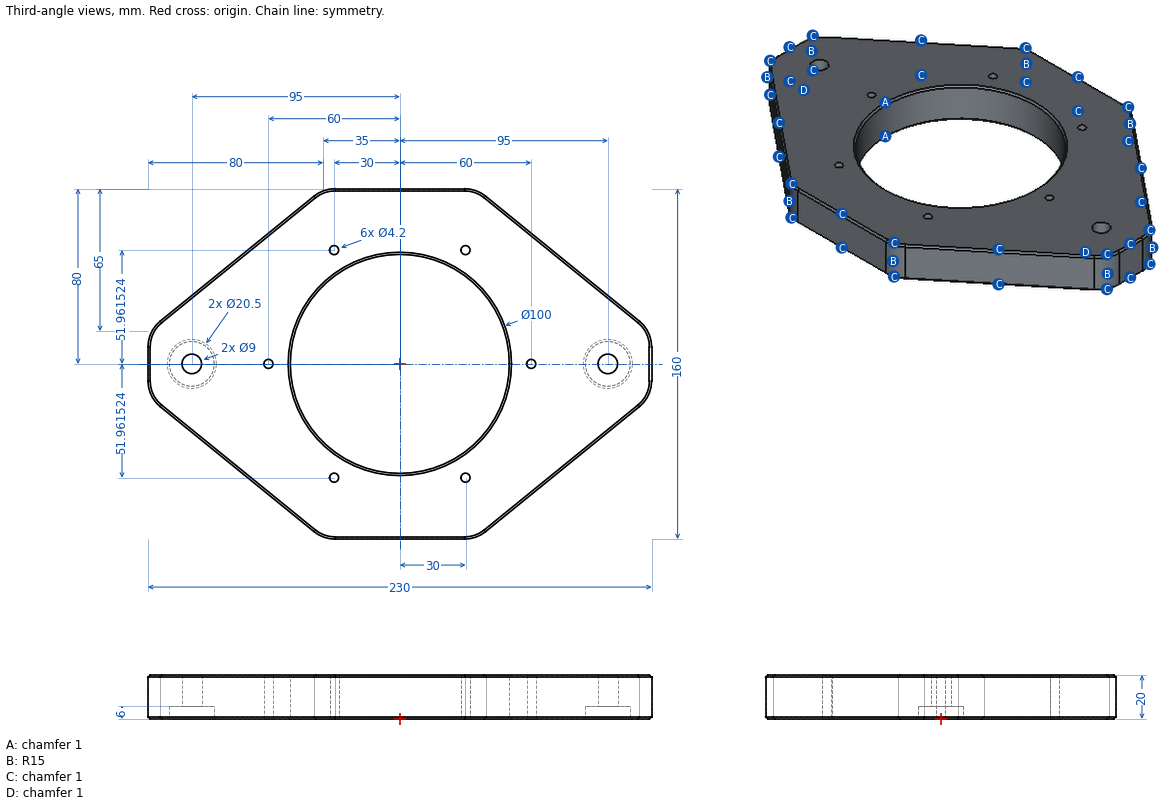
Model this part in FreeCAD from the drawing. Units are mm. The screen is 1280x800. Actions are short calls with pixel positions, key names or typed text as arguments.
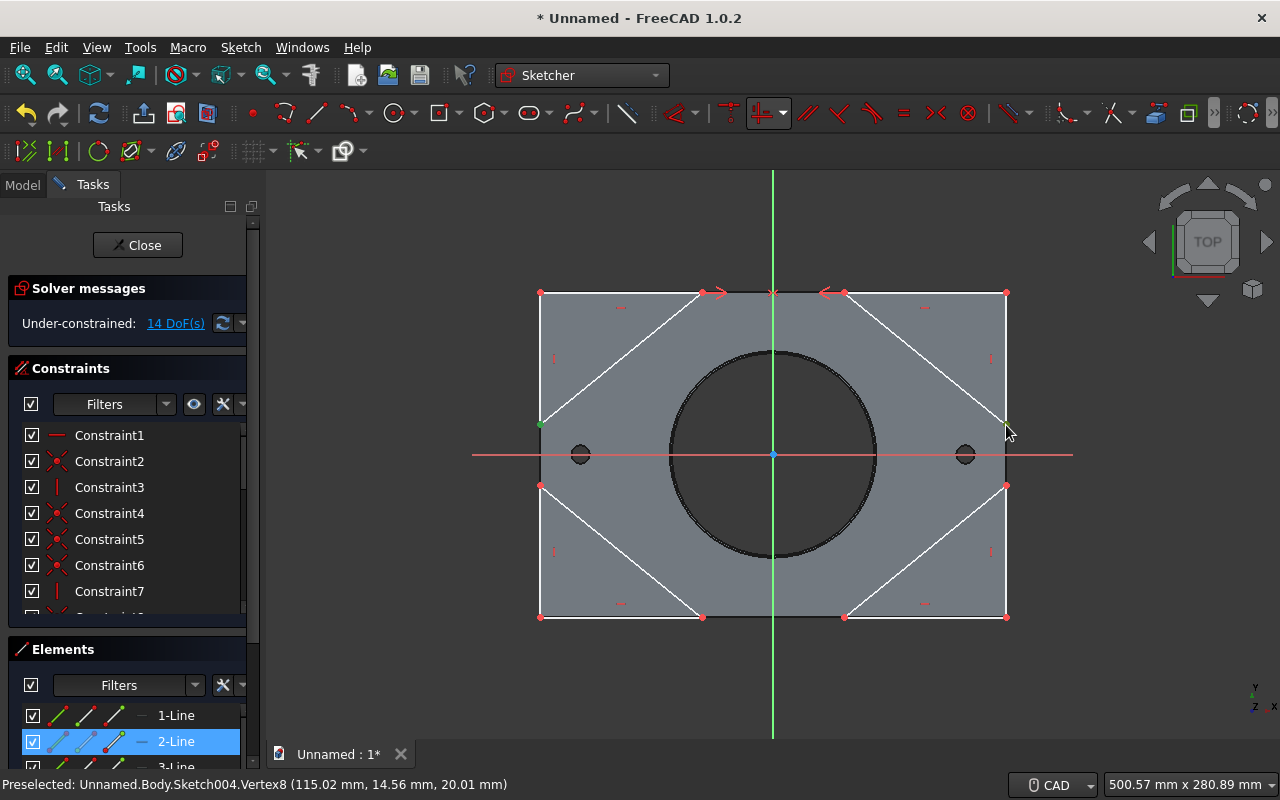
click(773, 674)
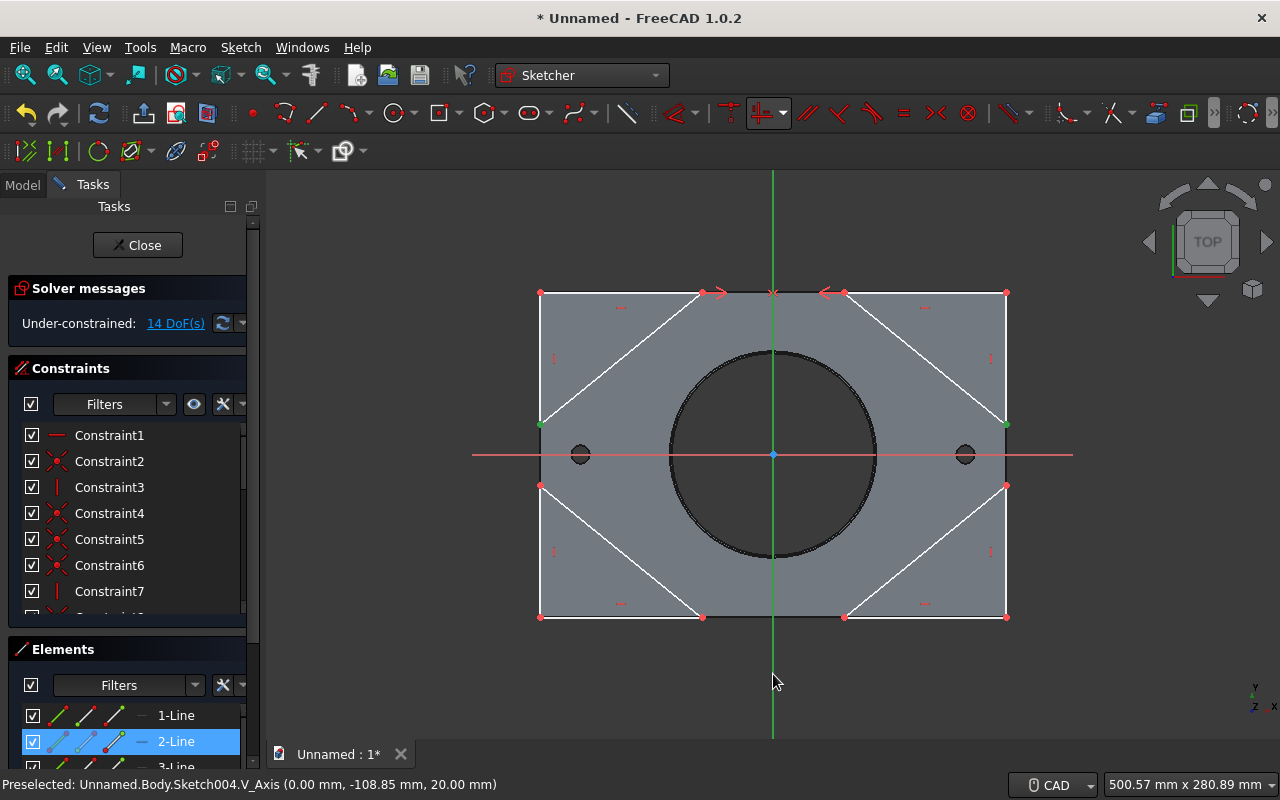
click(936, 114)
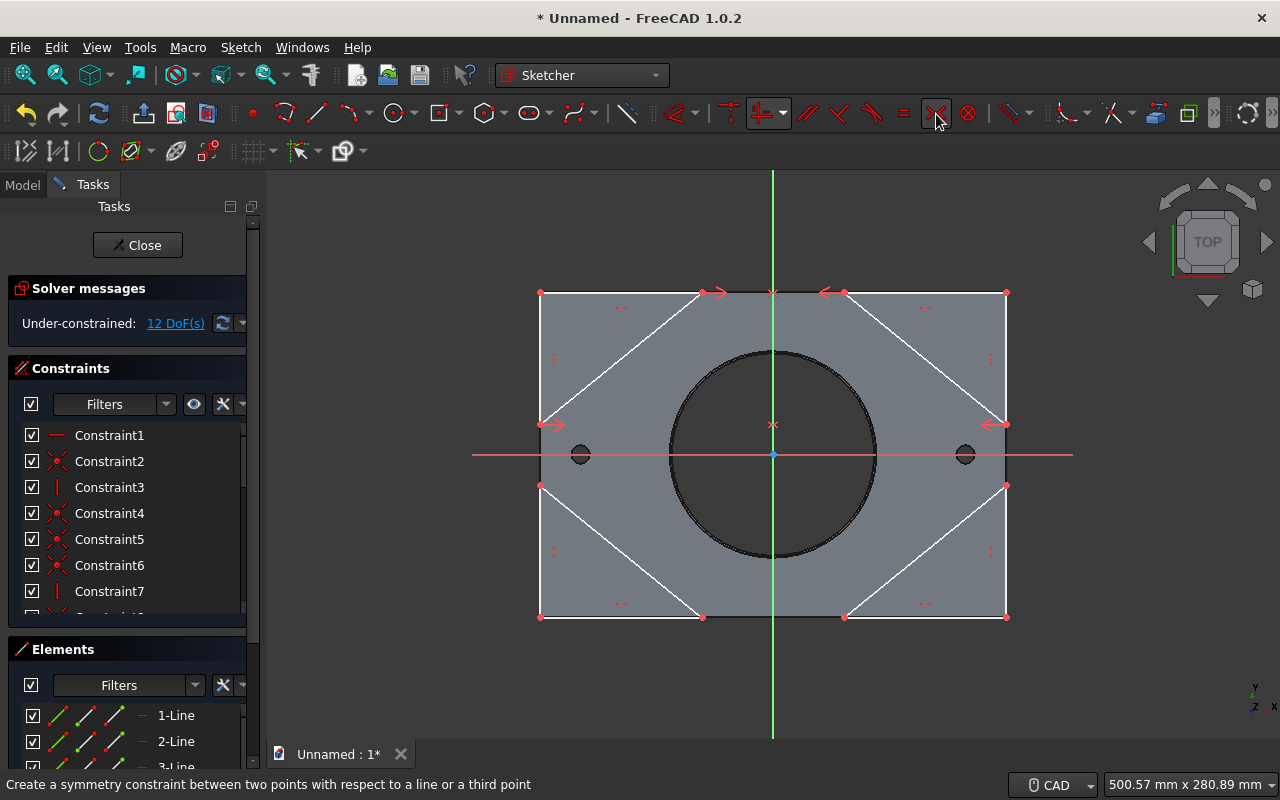
click(702, 293)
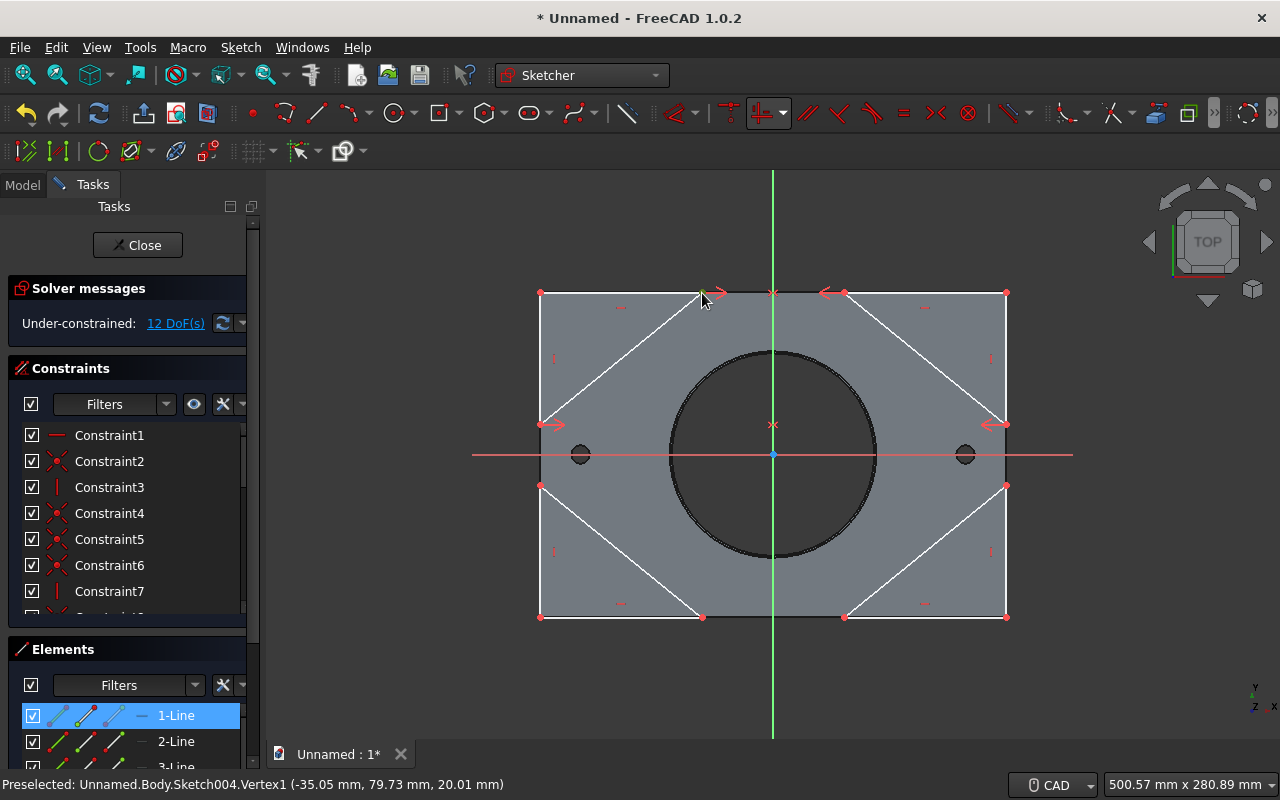
click(702, 618)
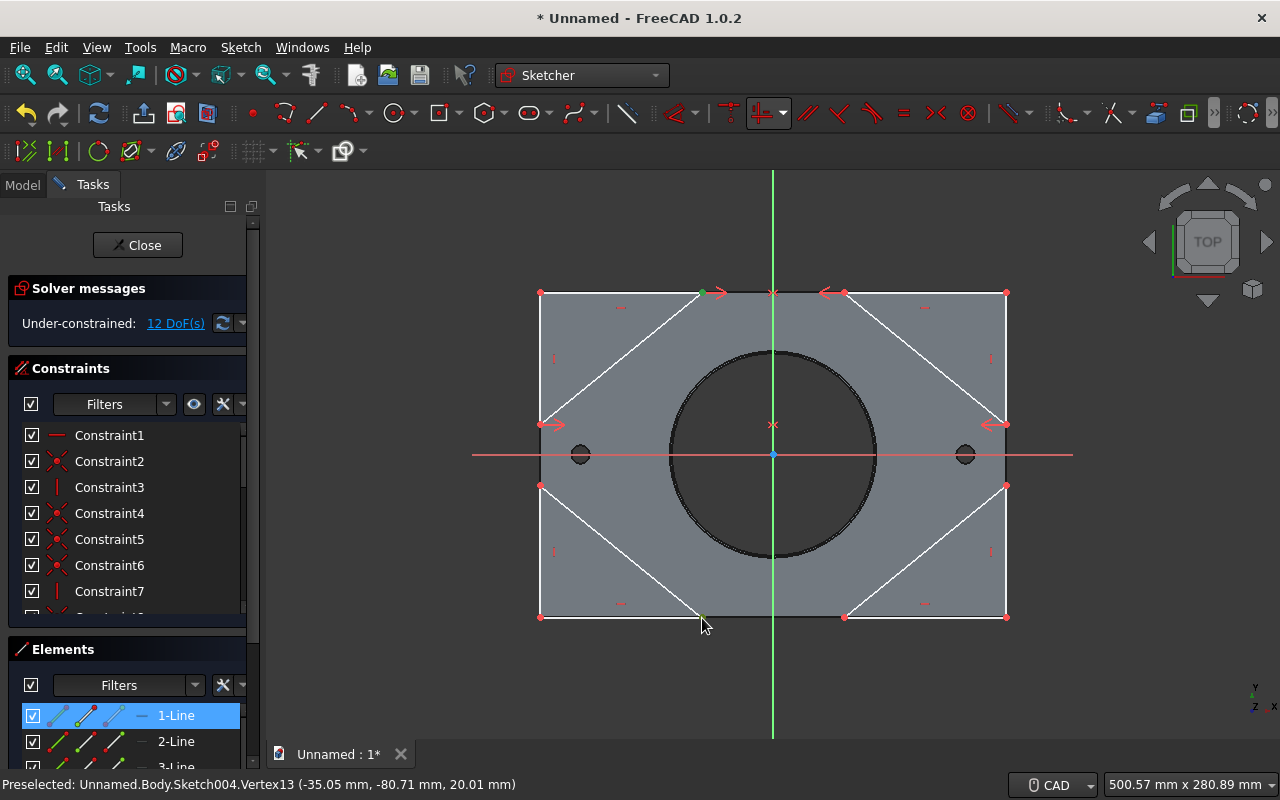
click(470, 454)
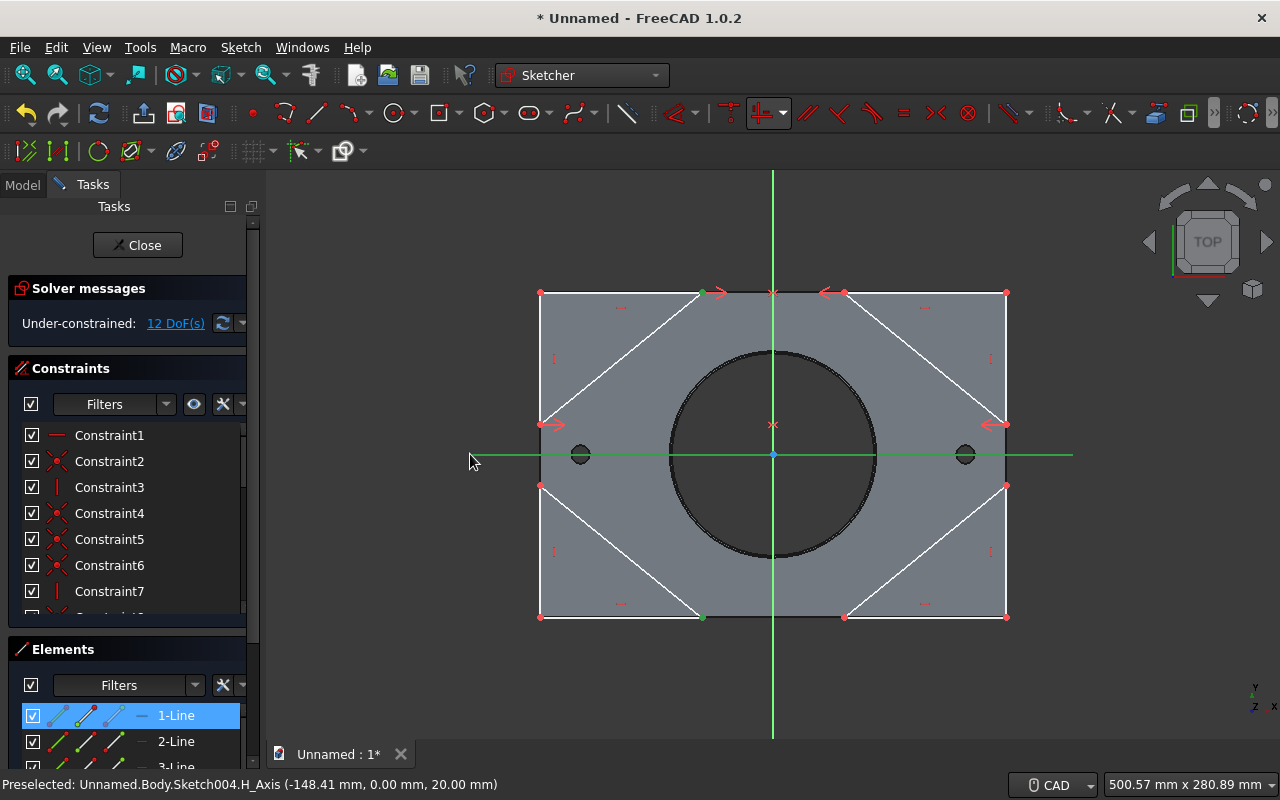
click(936, 114)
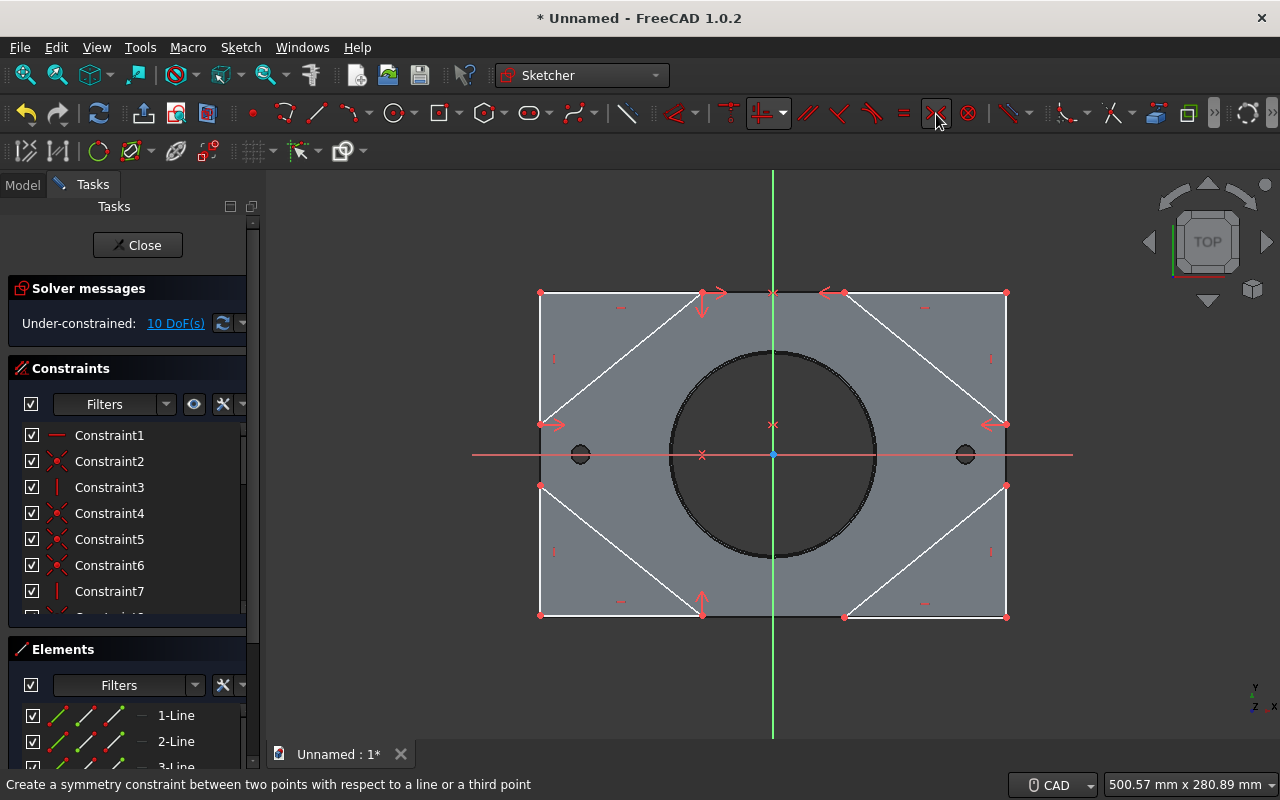
click(540, 425)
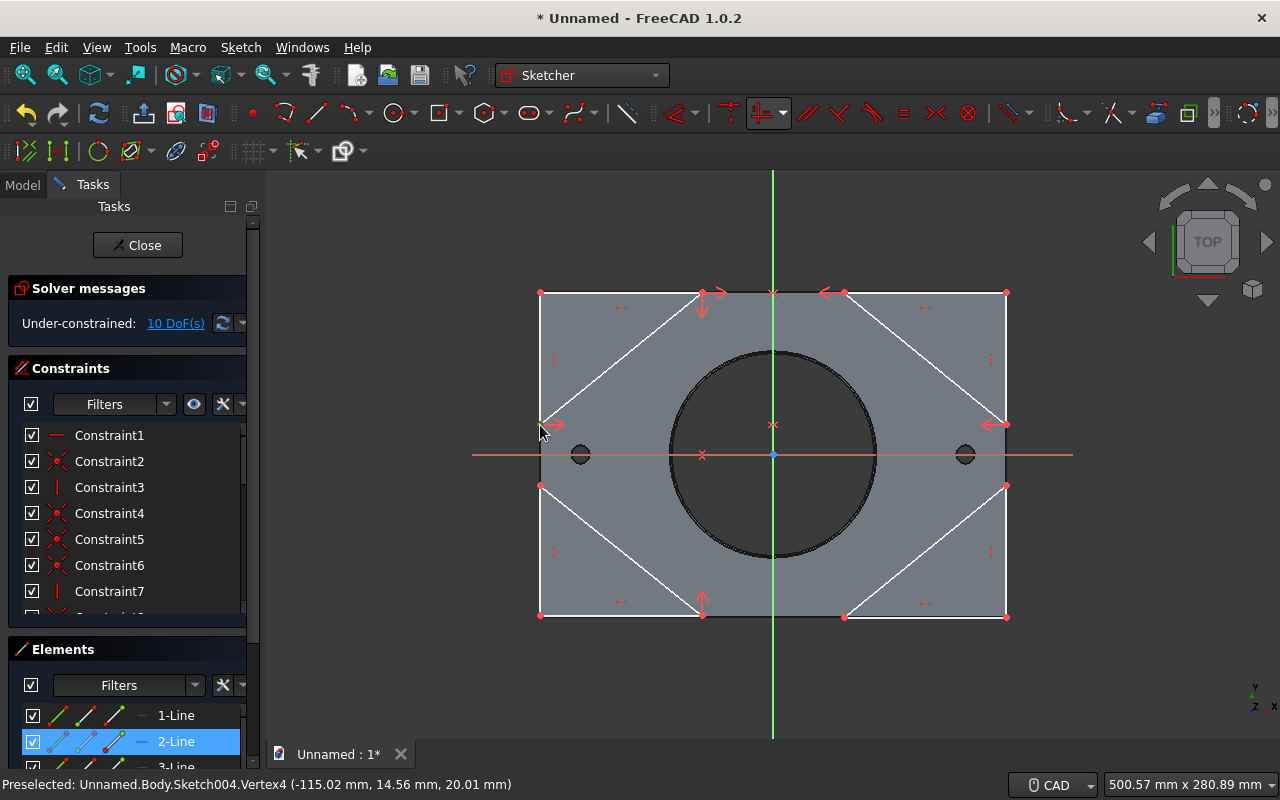
click(540, 486)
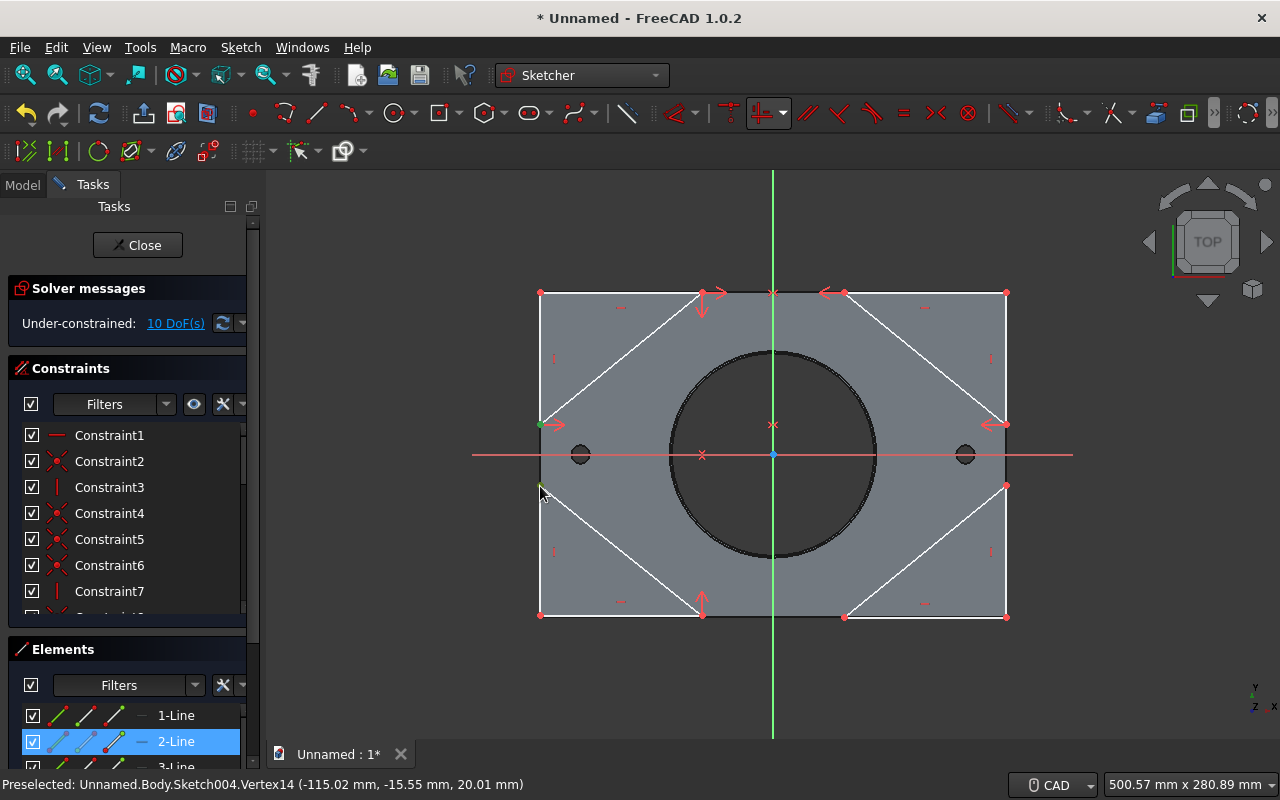
click(470, 454)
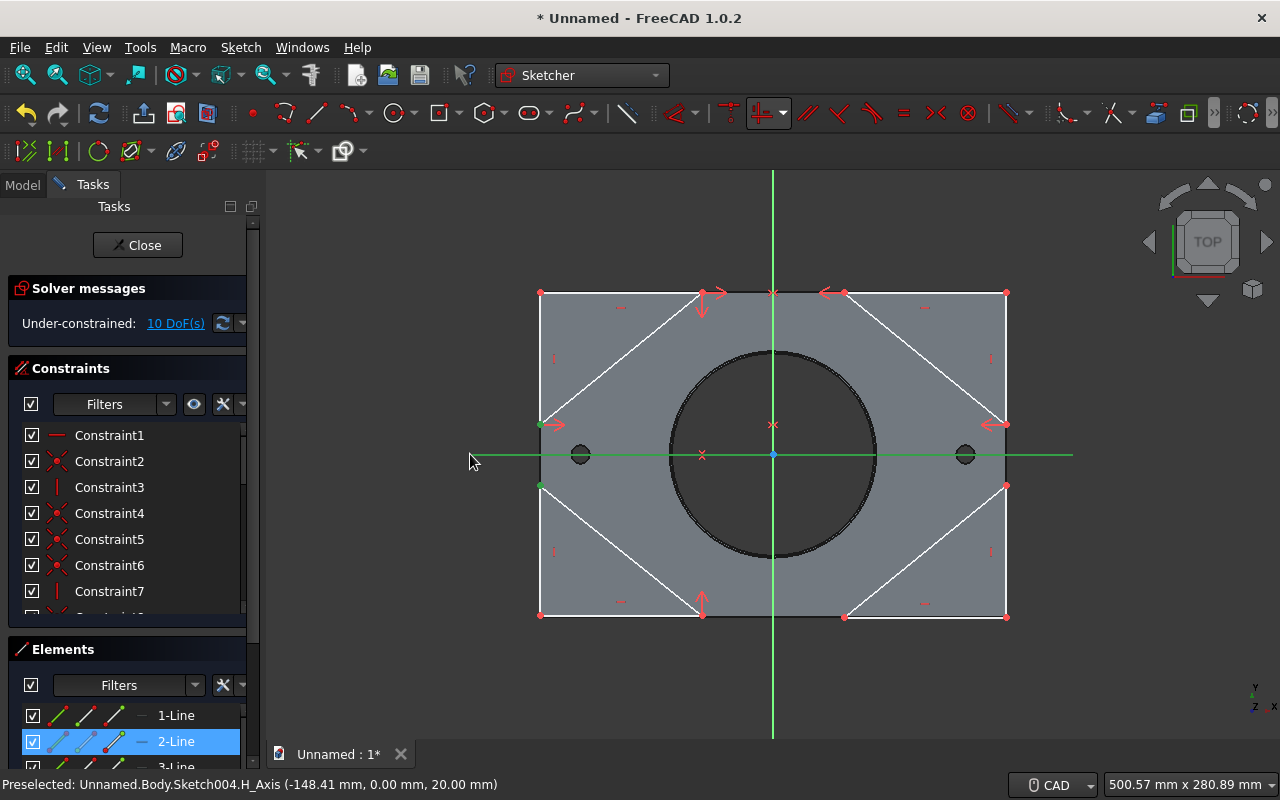
click(936, 114)